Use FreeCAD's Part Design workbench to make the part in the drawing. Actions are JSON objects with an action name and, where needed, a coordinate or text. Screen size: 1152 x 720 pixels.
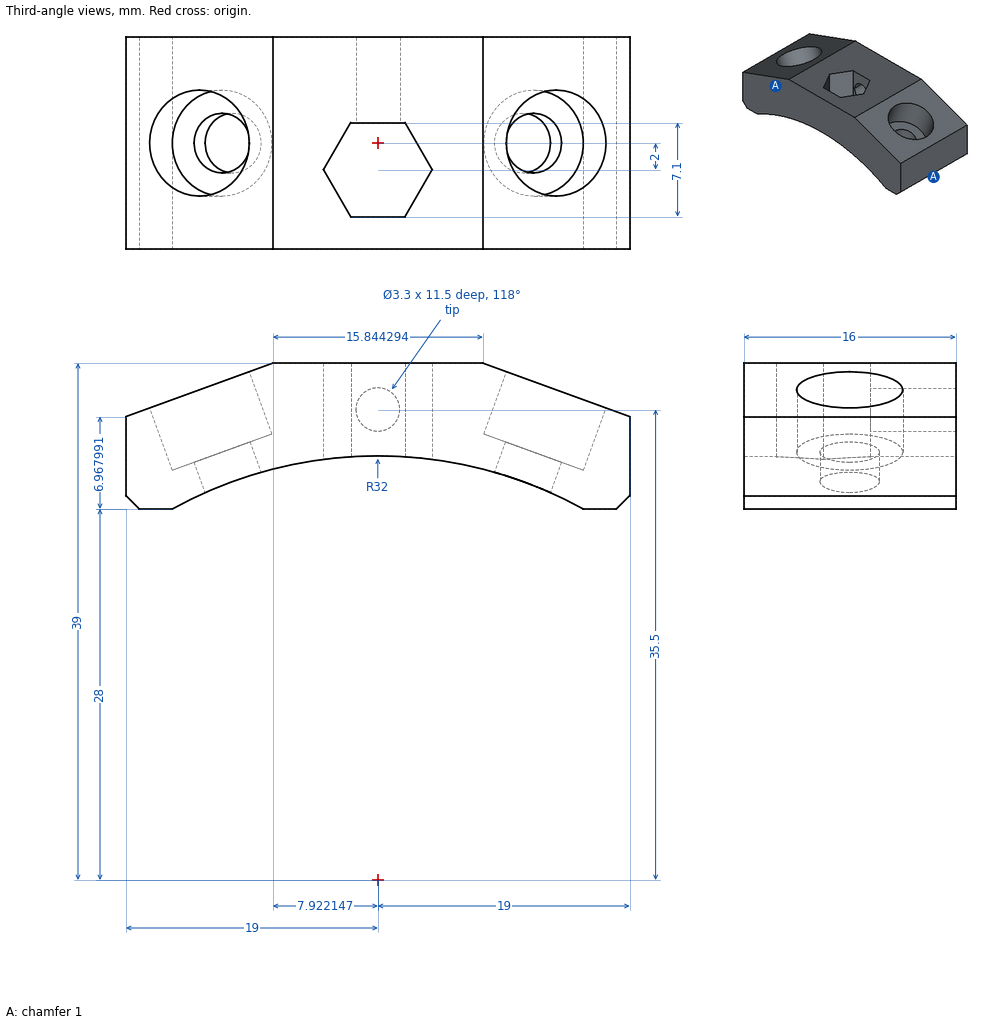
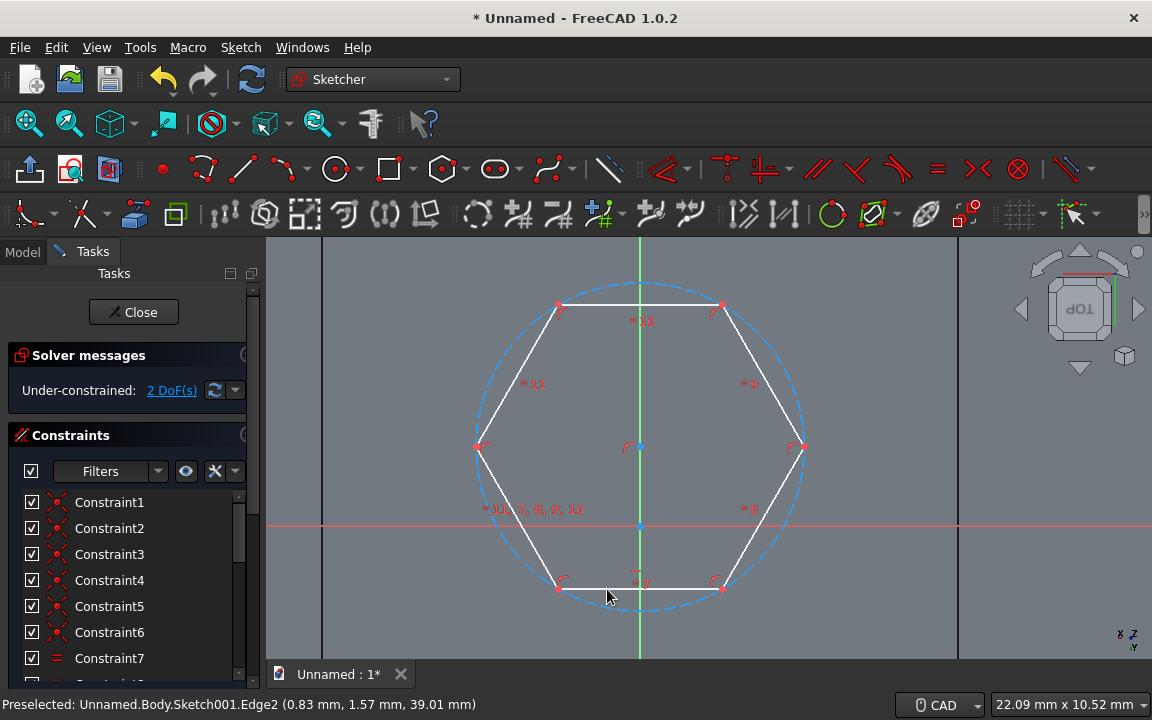
{"action": "left_click", "coordinate": [664, 170]}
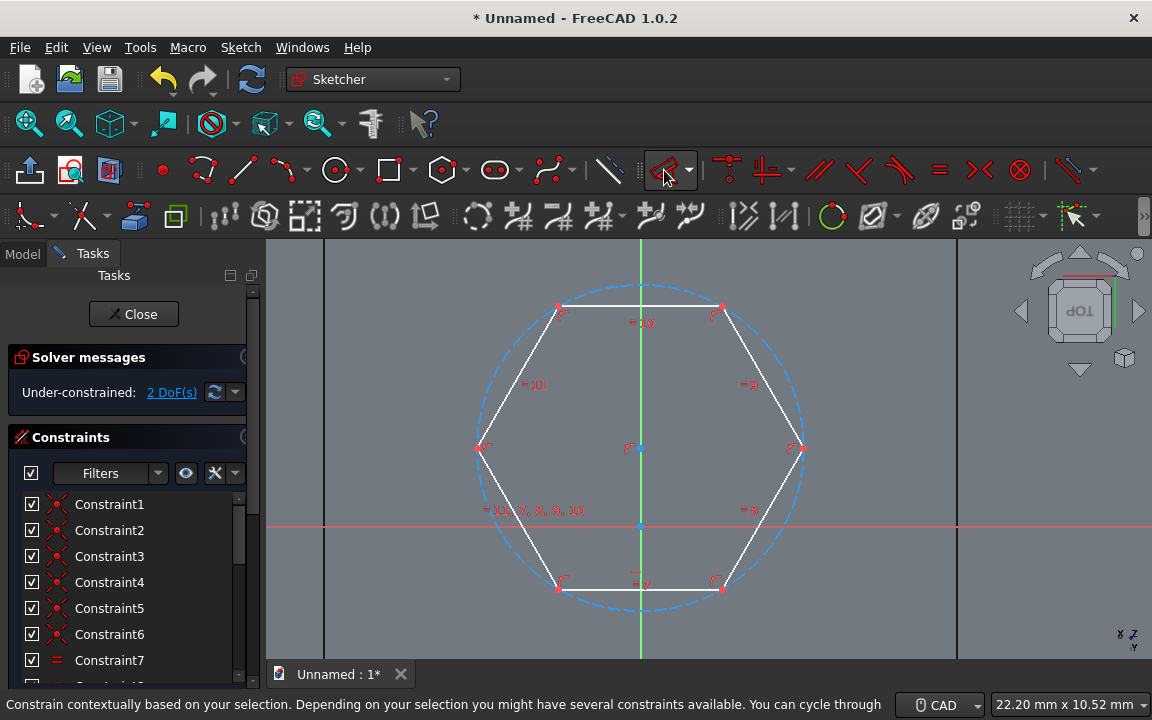
{"action": "left_click", "coordinate": [641, 448]}
{"action": "left_click", "coordinate": [675, 487]}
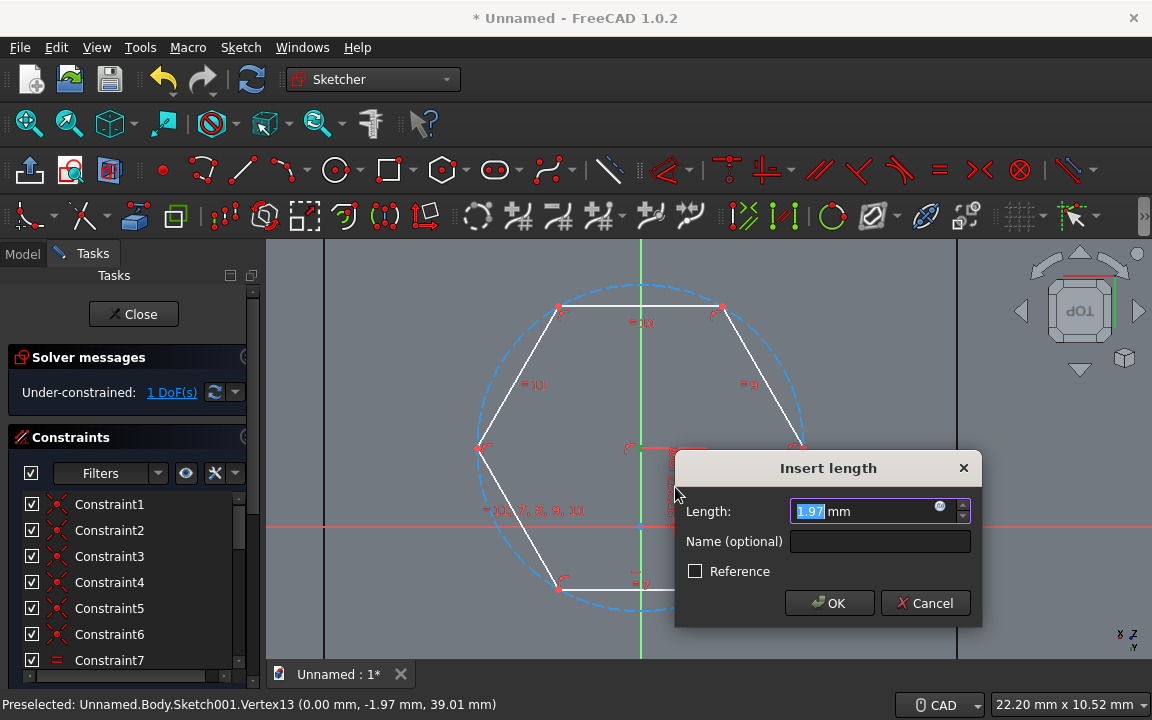
{"action": "type", "text": "2"}
{"action": "key", "text": "Return"}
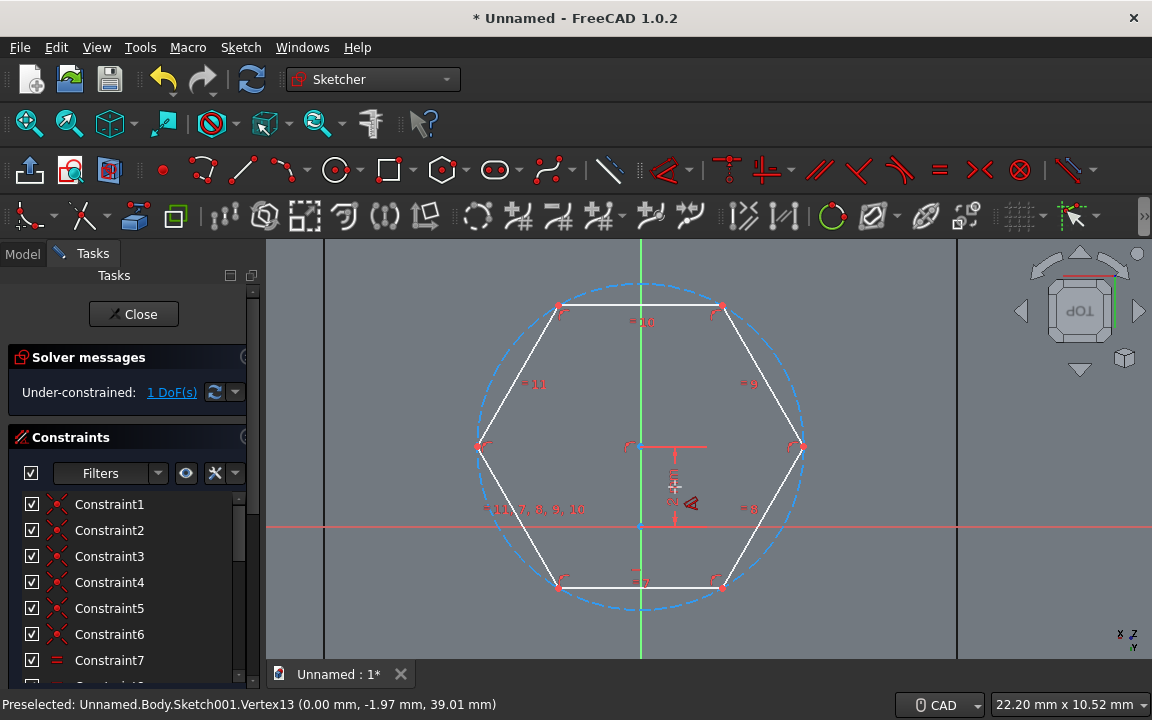
{"action": "left_click", "coordinate": [559, 588]}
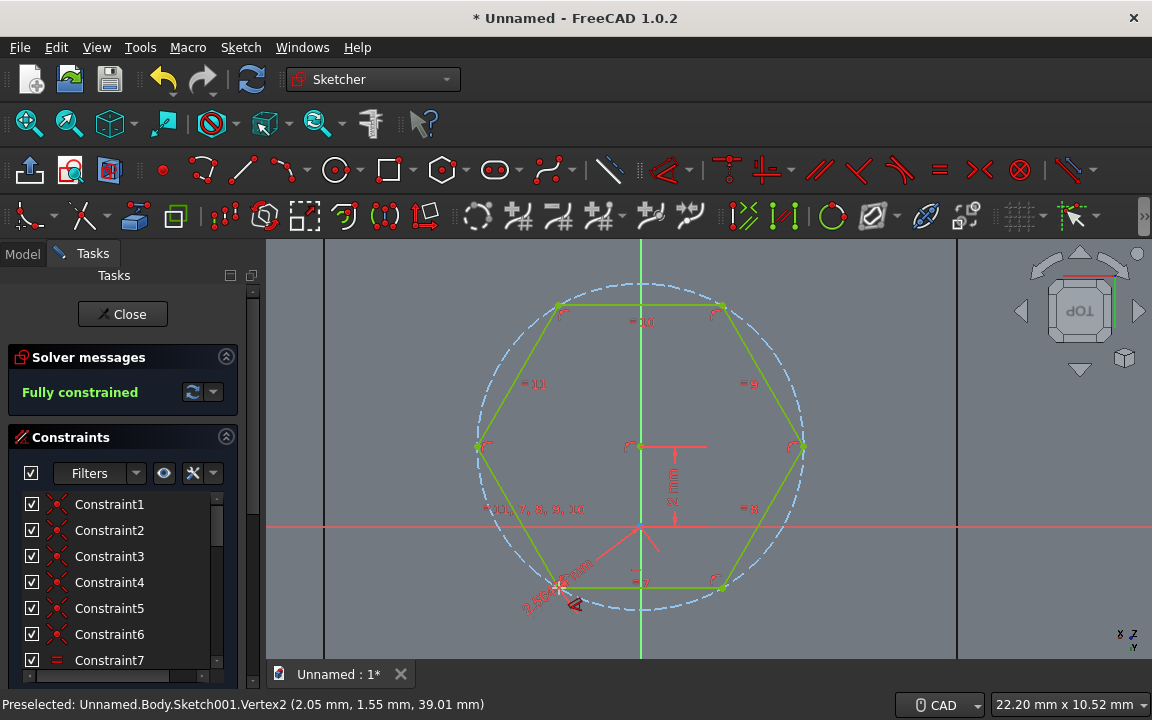
{"action": "left_click", "coordinate": [722, 305]}
{"action": "left_click", "coordinate": [525, 447]}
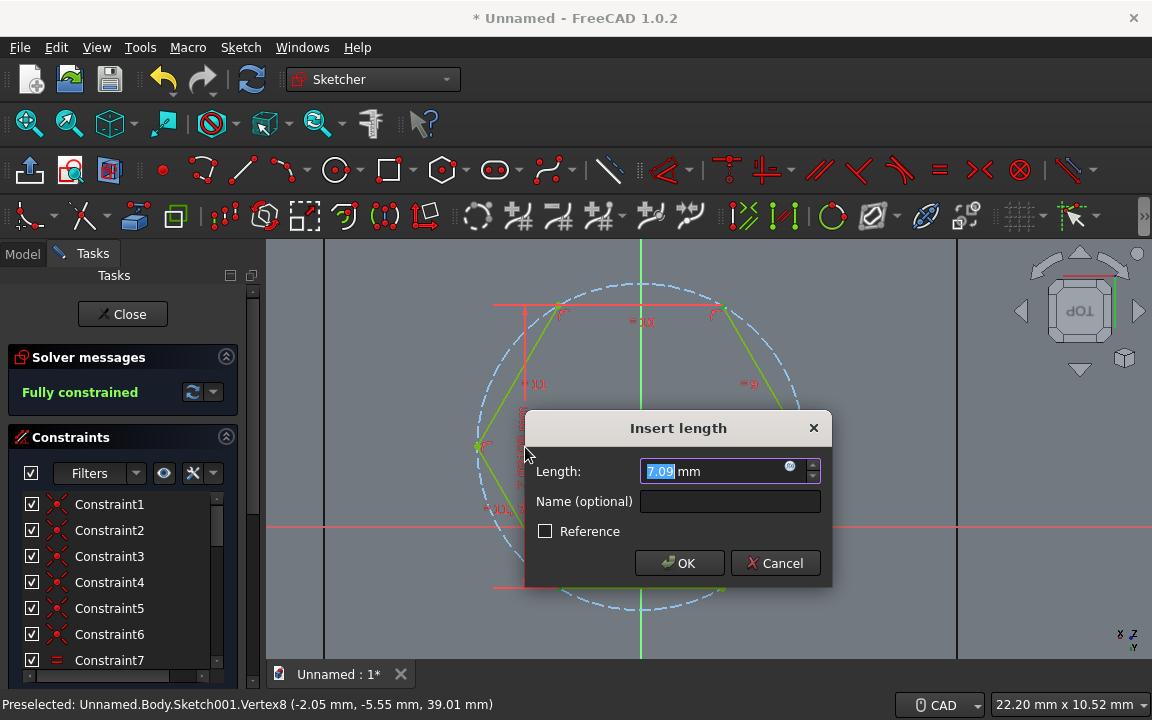
{"action": "type", "text": "7.1"}
{"action": "key", "text": "Return"}
{"action": "key", "text": "Escape"}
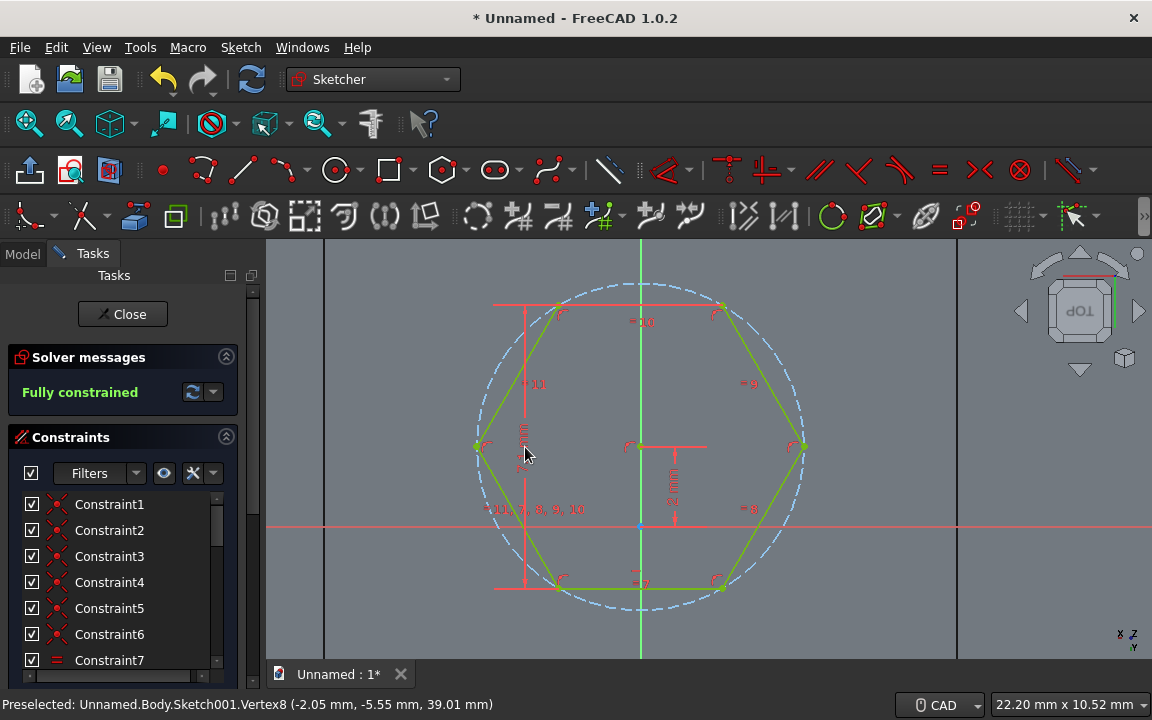
{"action": "left_click", "coordinate": [123, 314]}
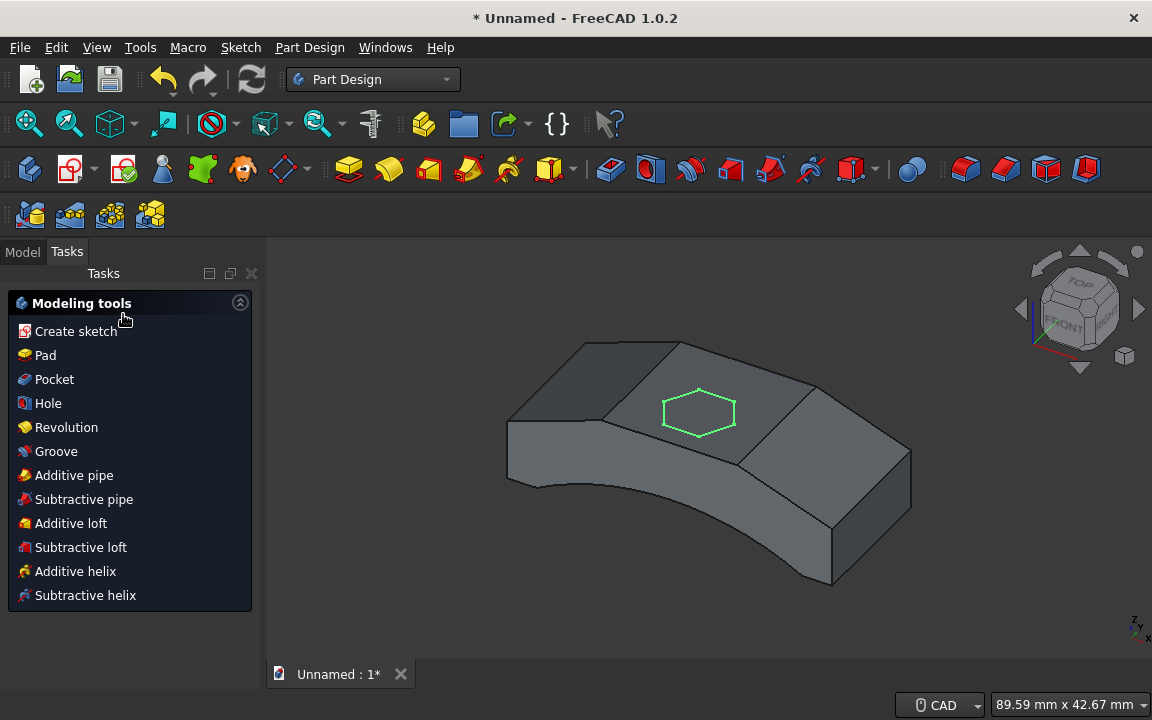
{"action": "left_click", "coordinate": [612, 170]}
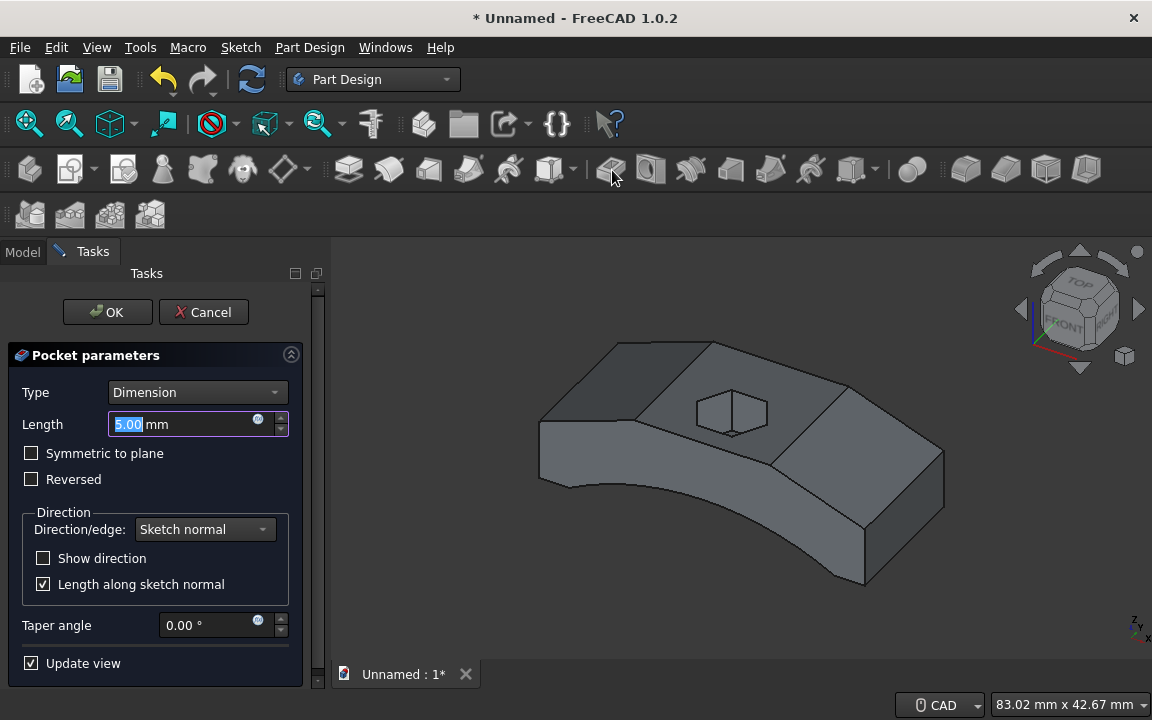
{"action": "left_click", "coordinate": [198, 392]}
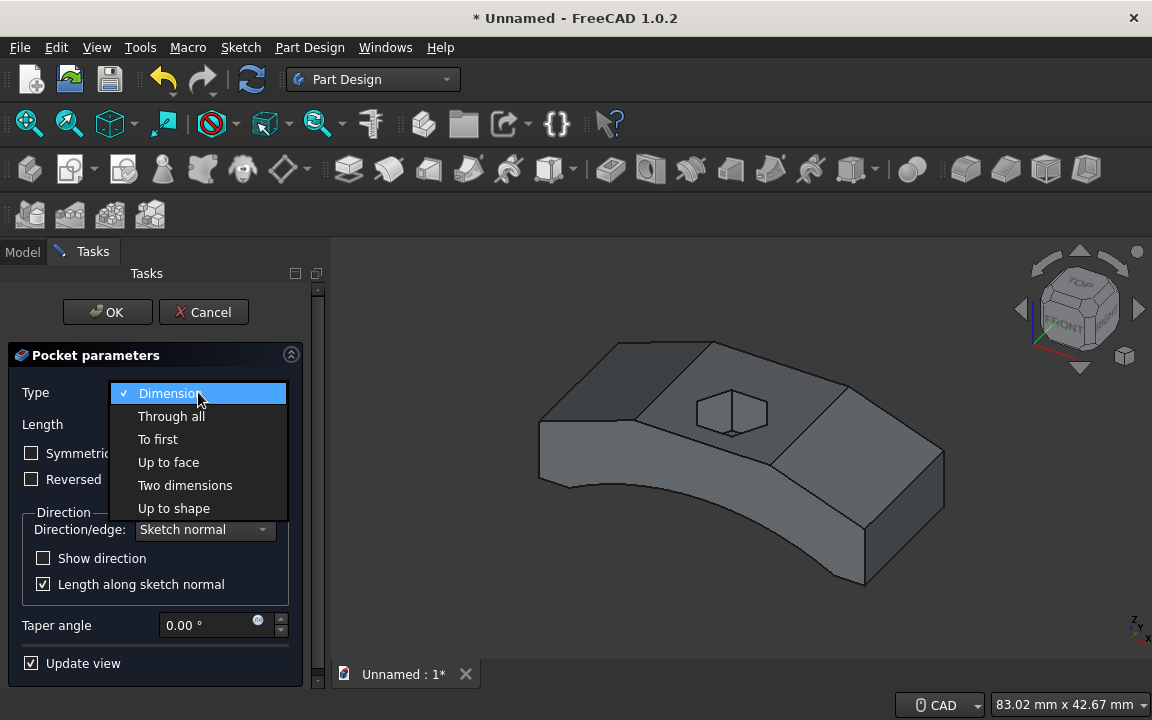
{"action": "left_click", "coordinate": [198, 416]}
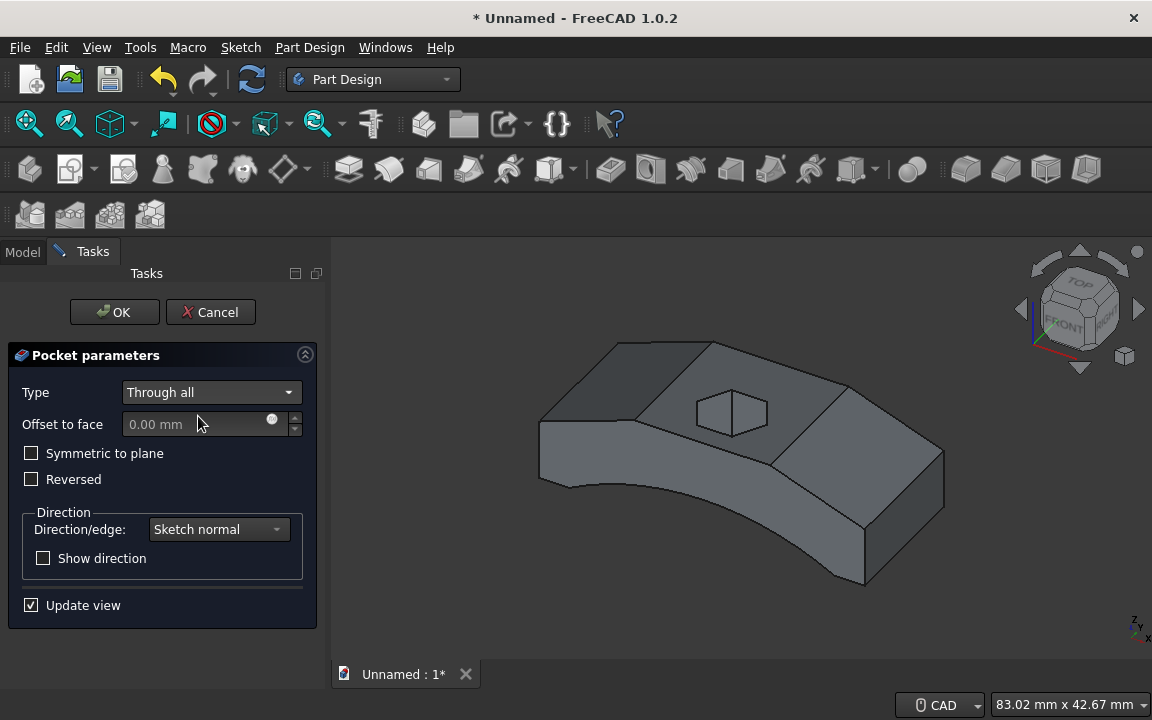
{"action": "left_click", "coordinate": [115, 312]}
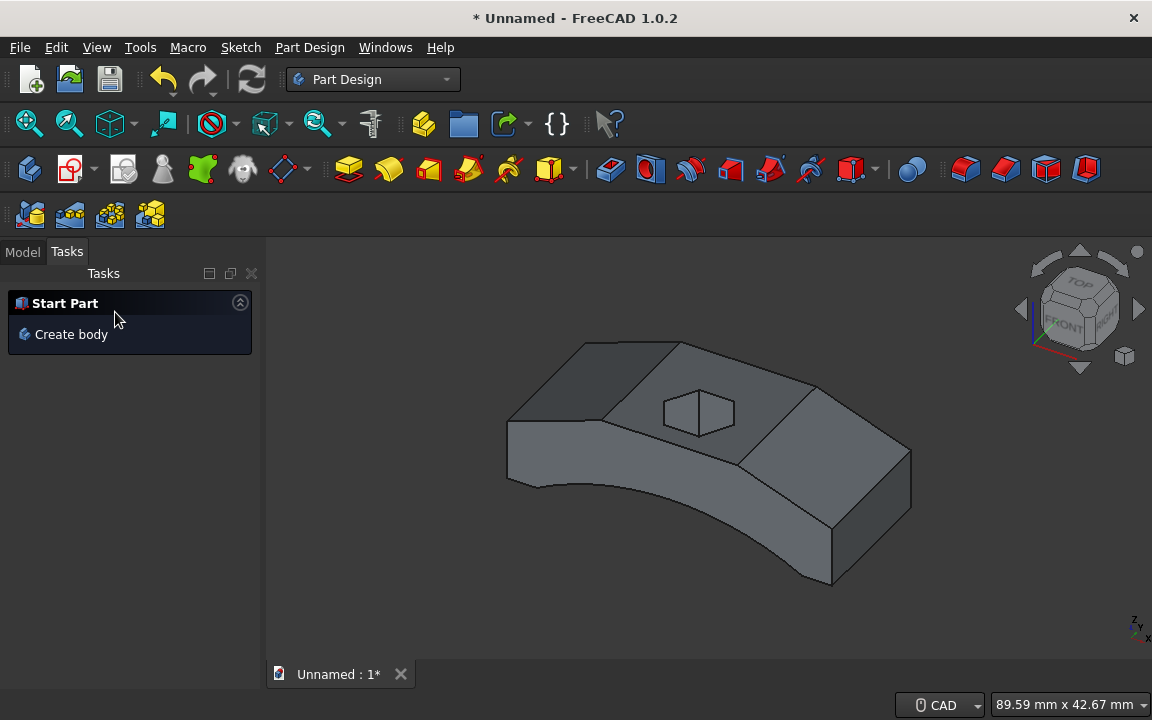
{"action": "key", "text": "4"}